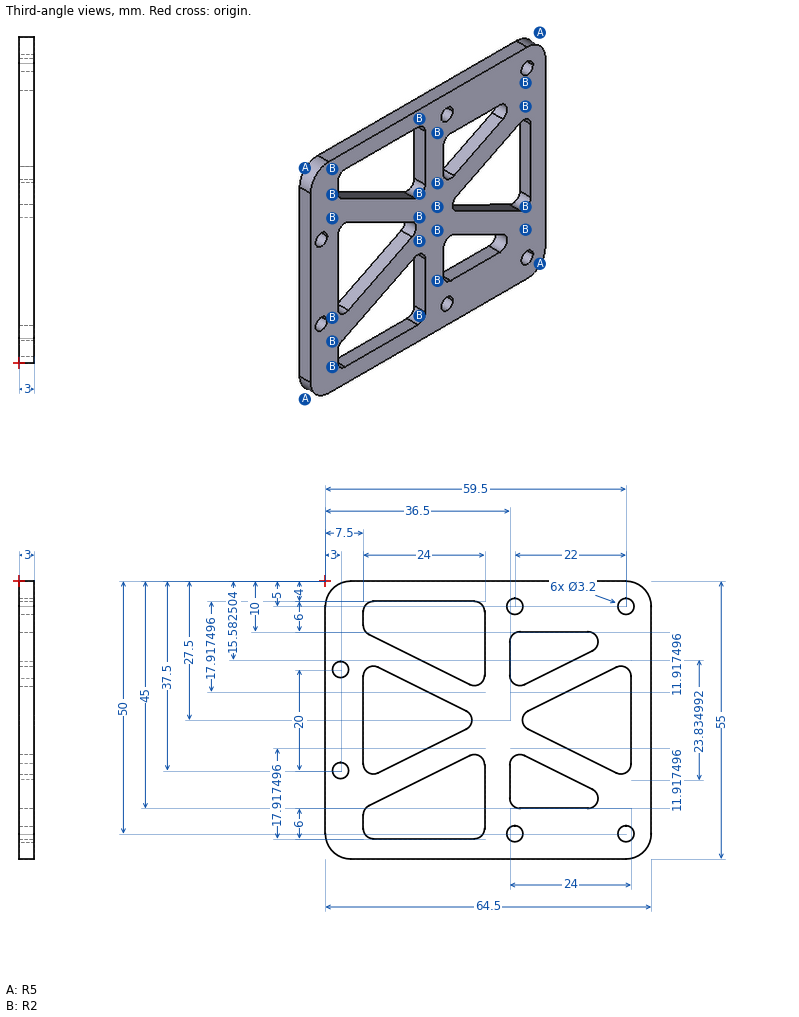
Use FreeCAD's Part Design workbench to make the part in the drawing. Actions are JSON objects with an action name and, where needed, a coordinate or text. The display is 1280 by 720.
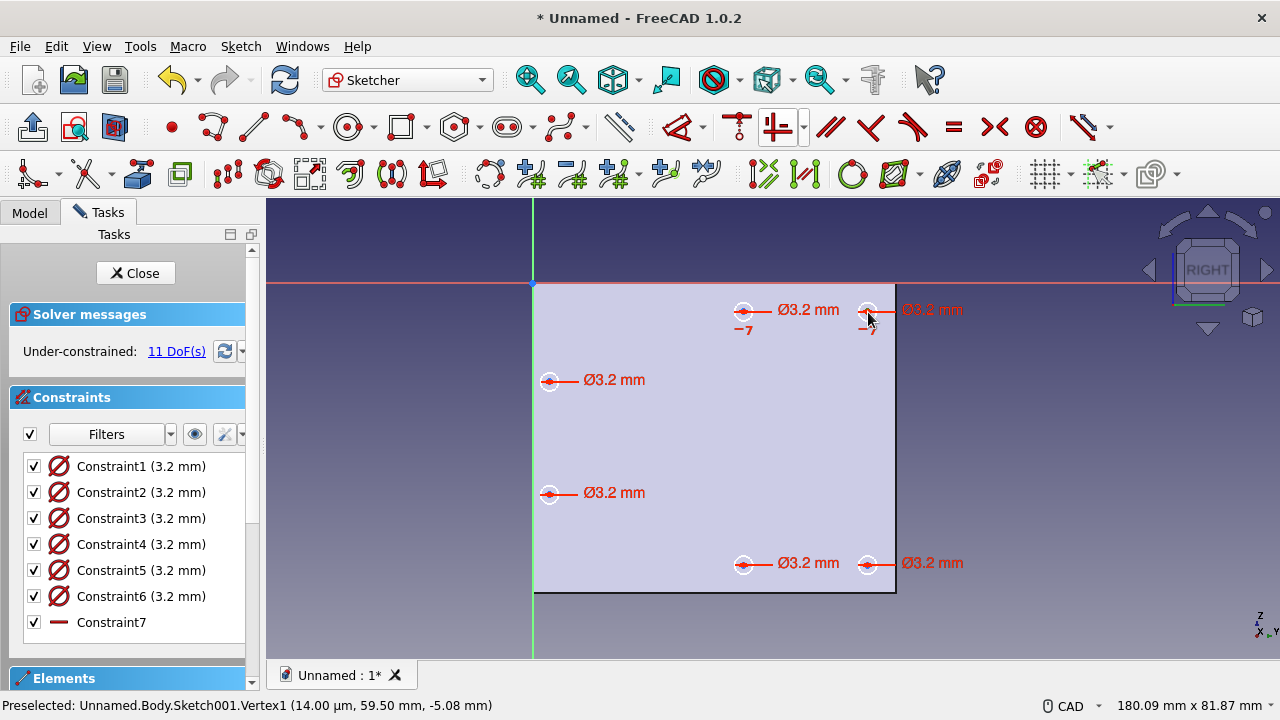
{"action": "left_click", "coordinate": [868, 565]}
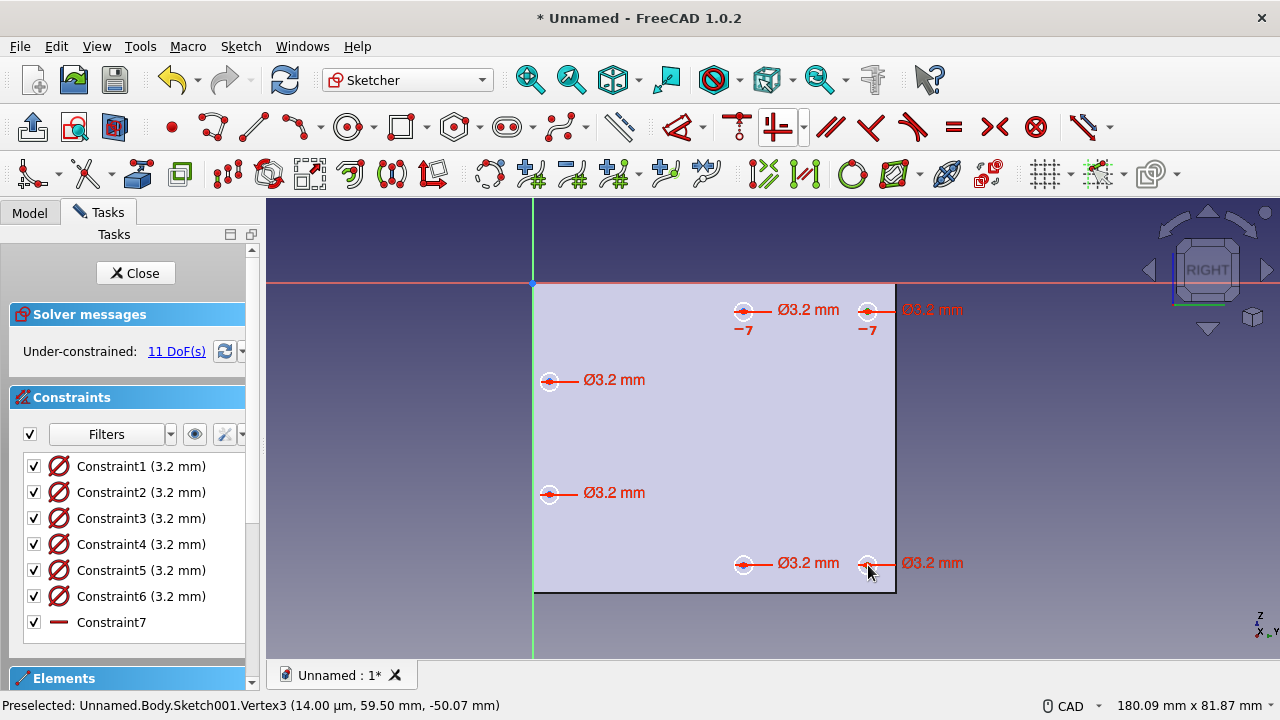
{"action": "left_click", "coordinate": [804, 128]}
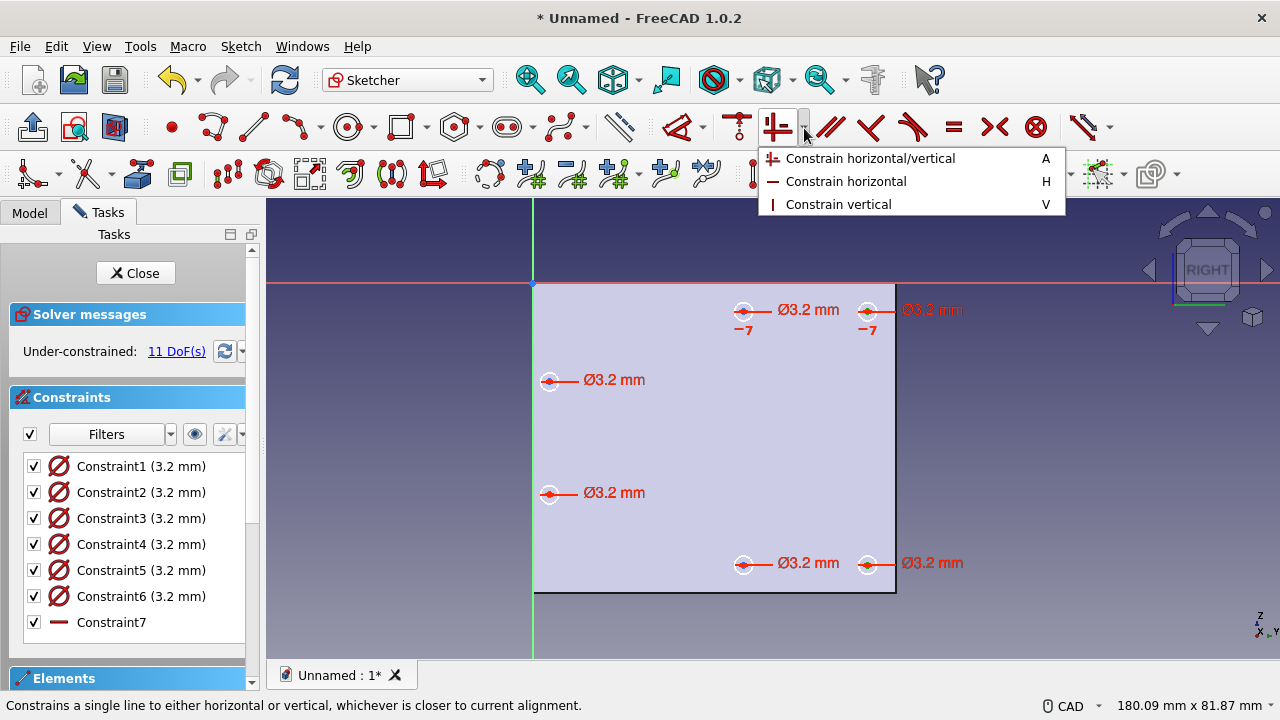
{"action": "left_click", "coordinate": [912, 204]}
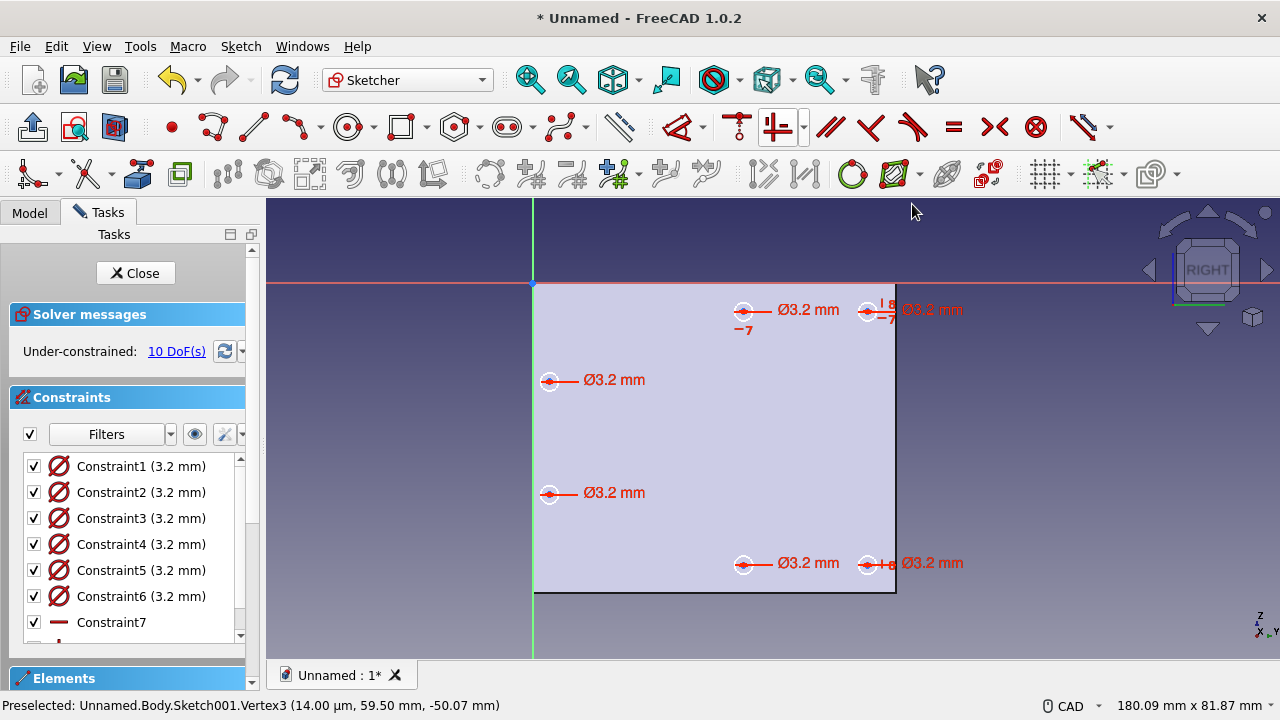
{"action": "left_click", "coordinate": [744, 312]}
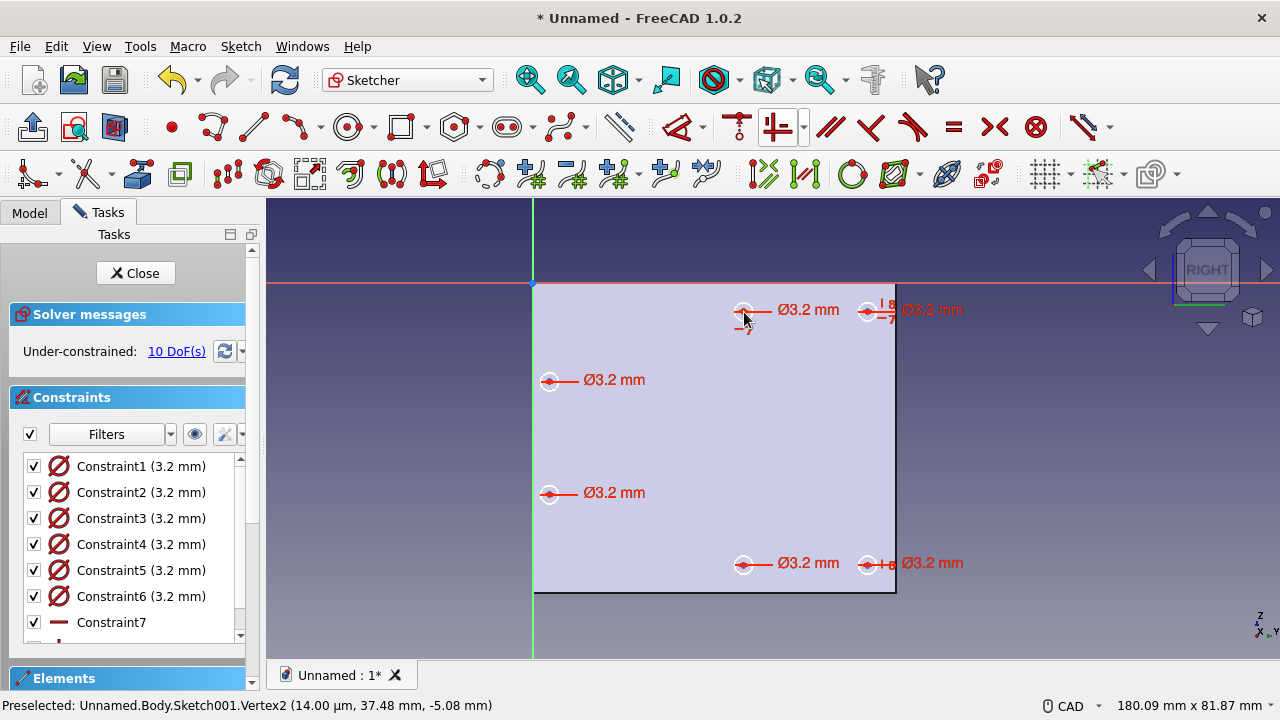
{"action": "left_click", "coordinate": [744, 565]}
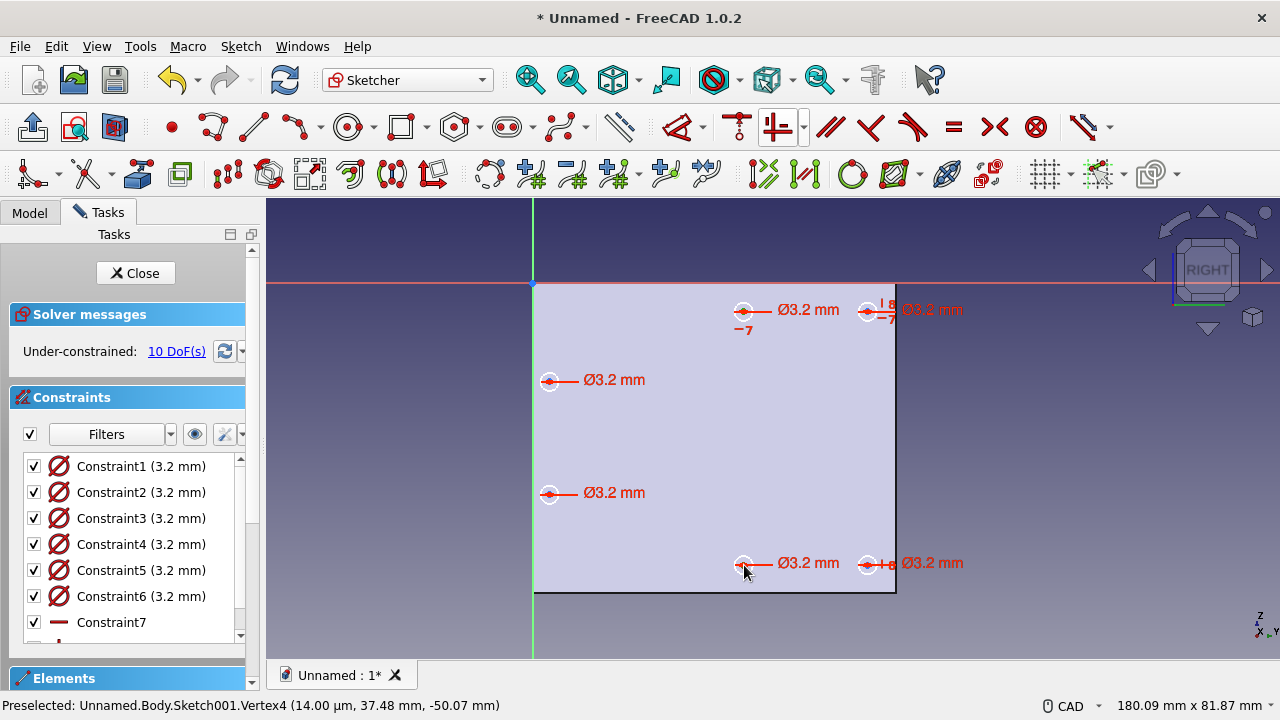
{"action": "left_click", "coordinate": [804, 128]}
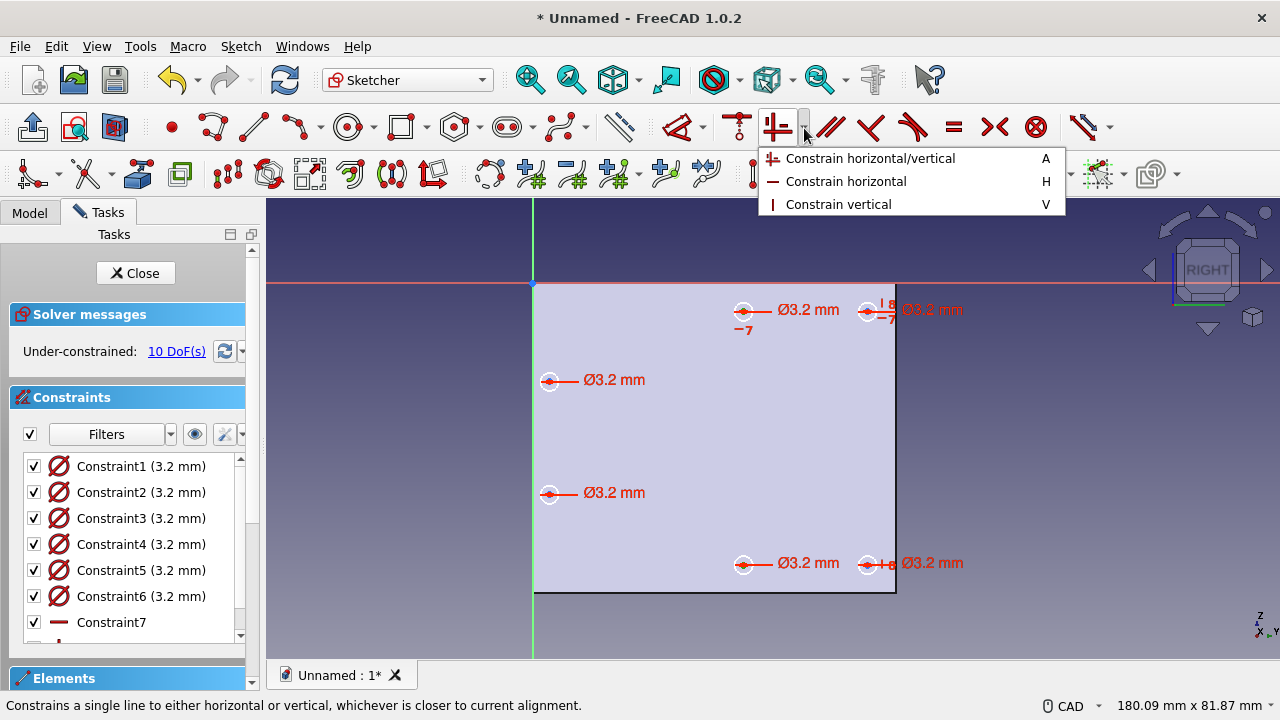
{"action": "left_click", "coordinate": [912, 204]}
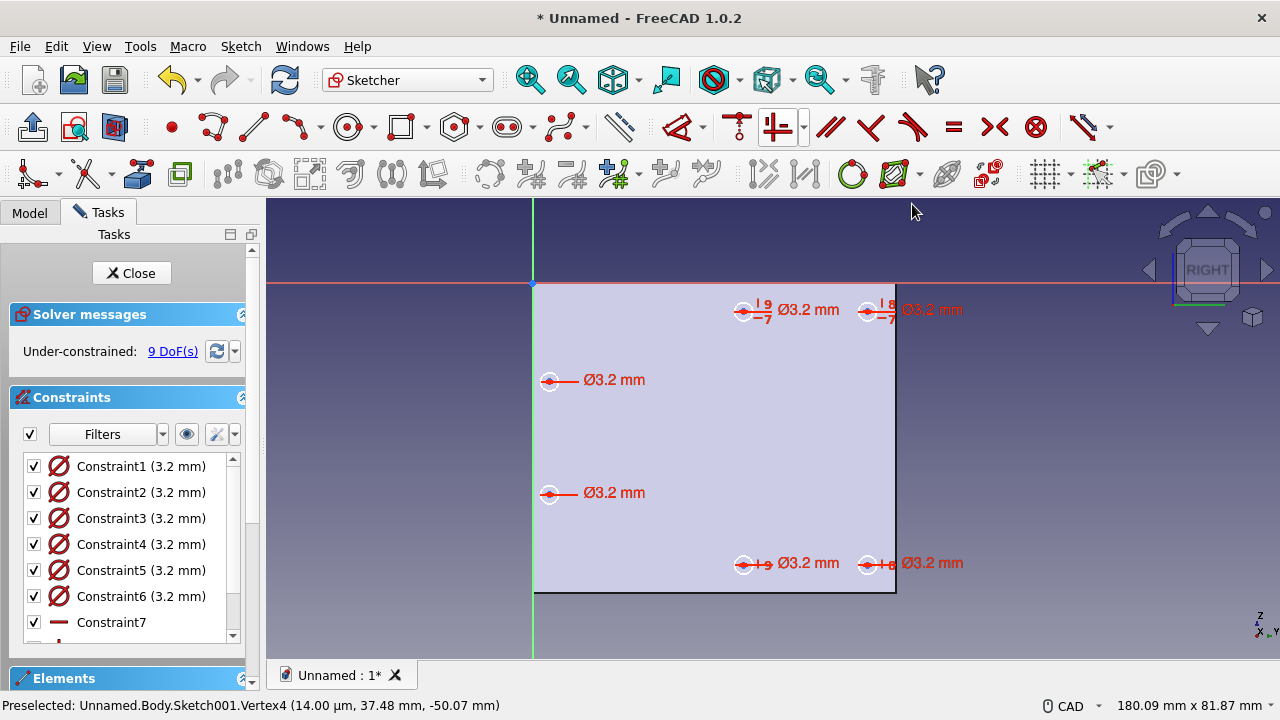
{"action": "left_click", "coordinate": [868, 565]}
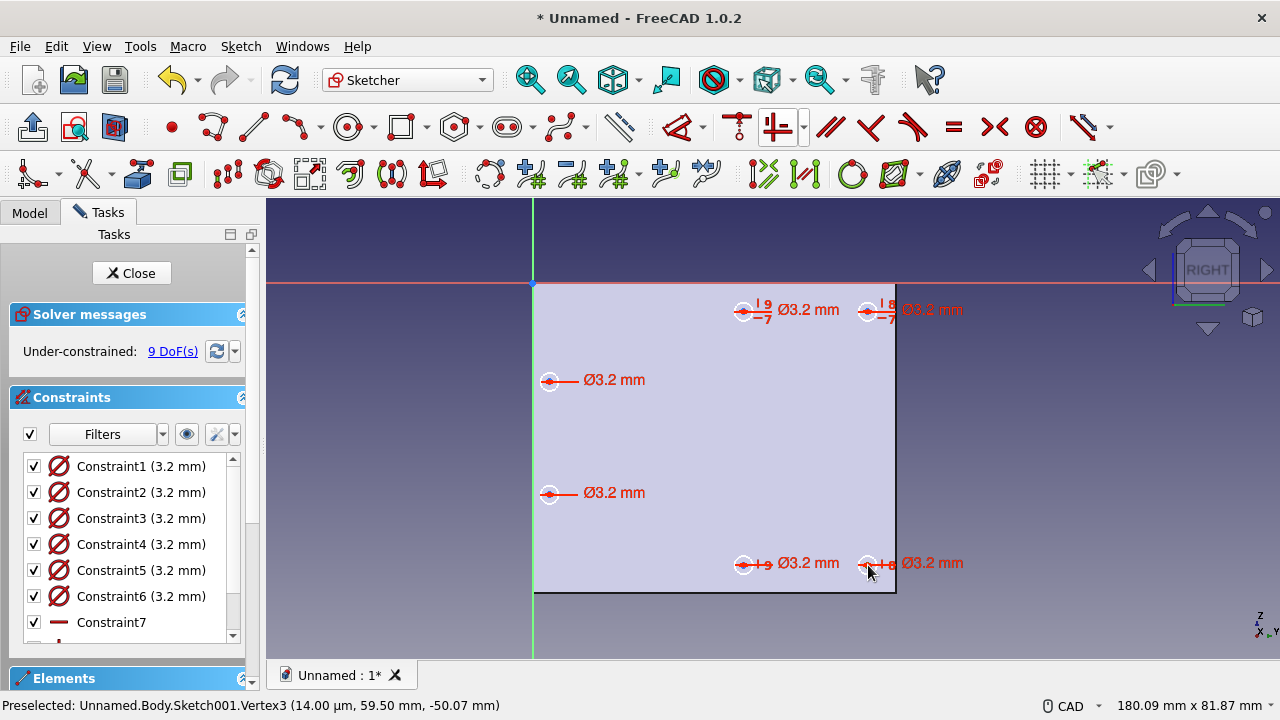
{"action": "left_click", "coordinate": [744, 565]}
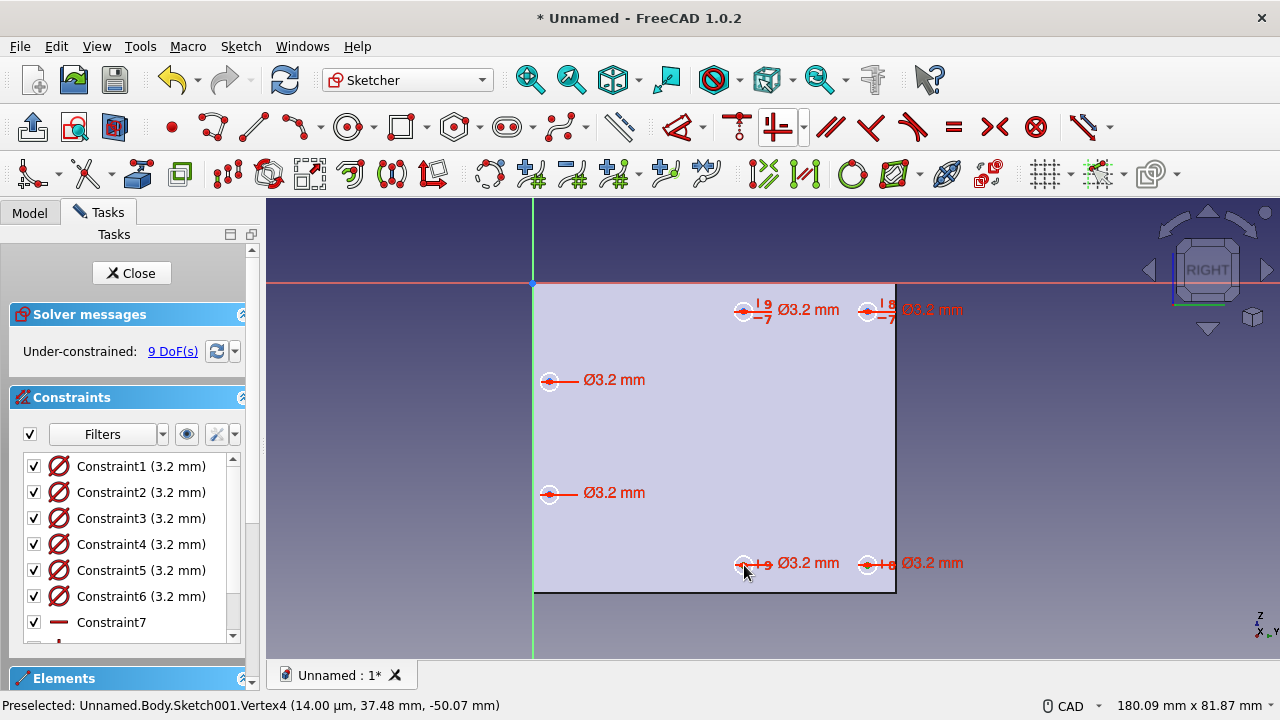
{"action": "left_click", "coordinate": [804, 128]}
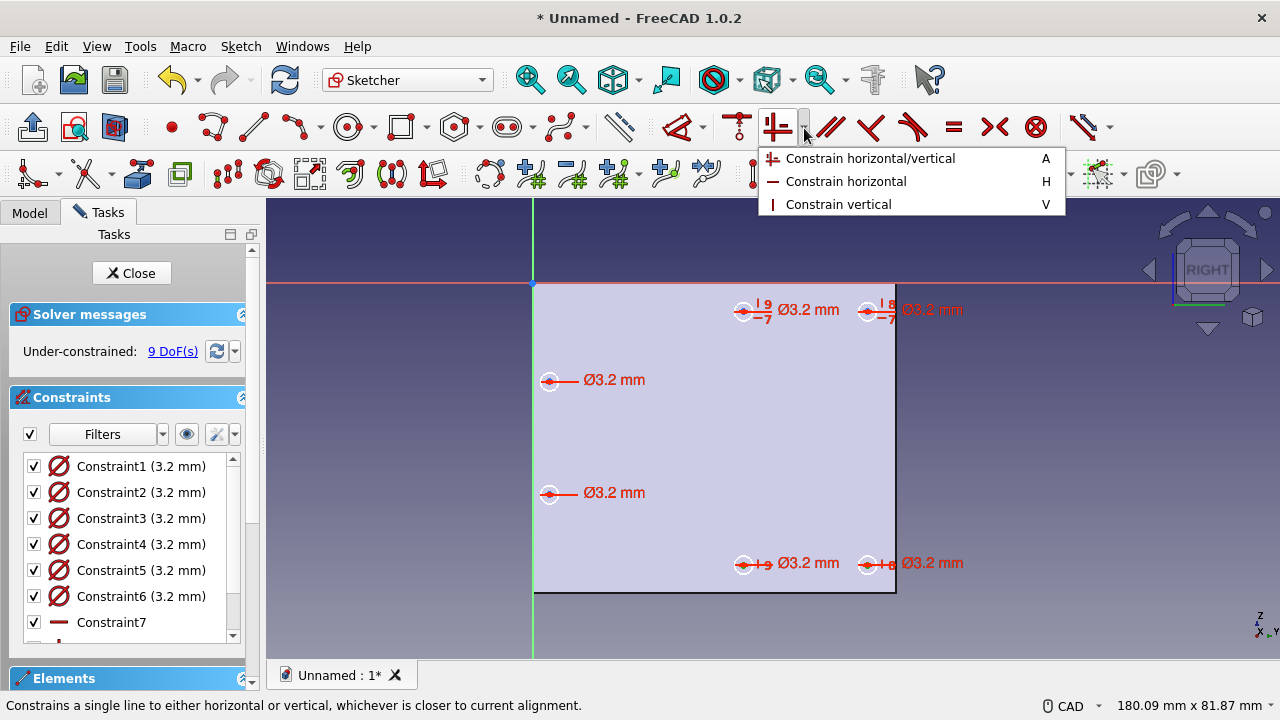
{"action": "left_click", "coordinate": [912, 182]}